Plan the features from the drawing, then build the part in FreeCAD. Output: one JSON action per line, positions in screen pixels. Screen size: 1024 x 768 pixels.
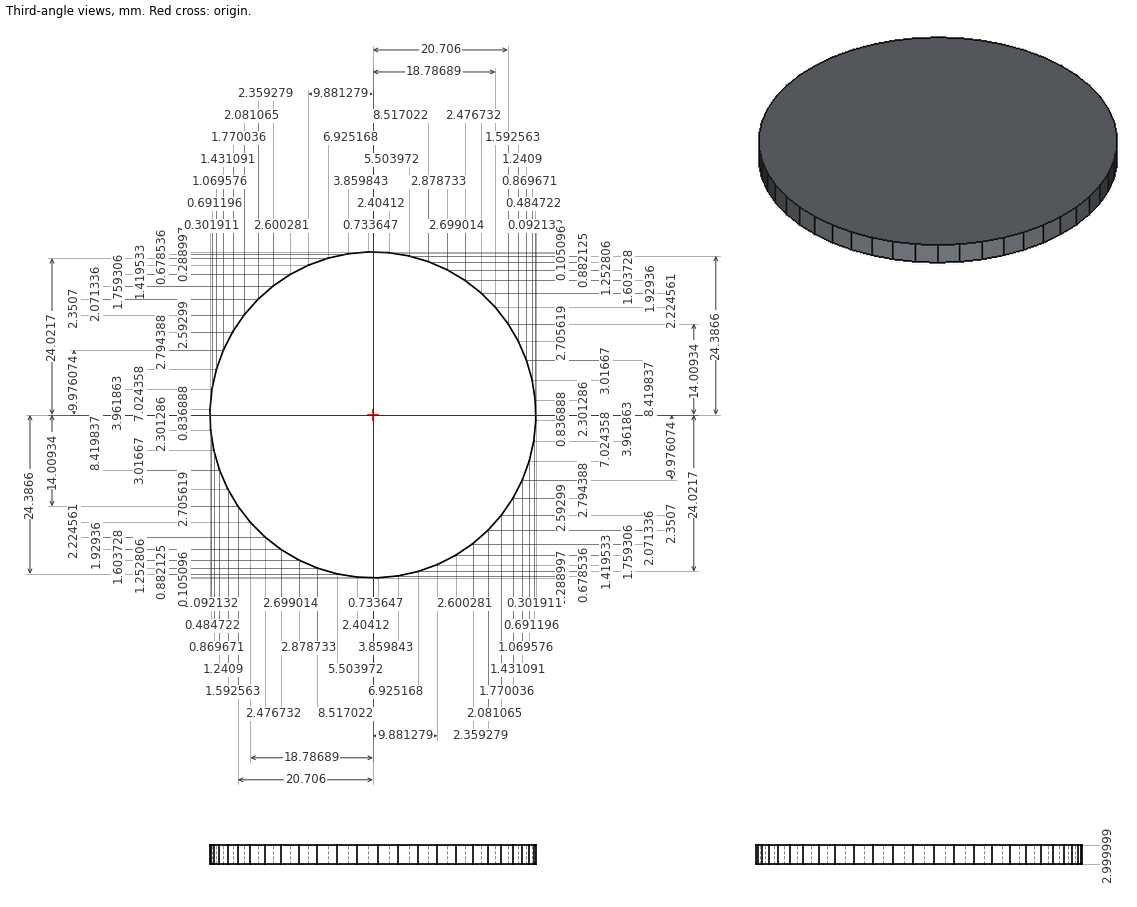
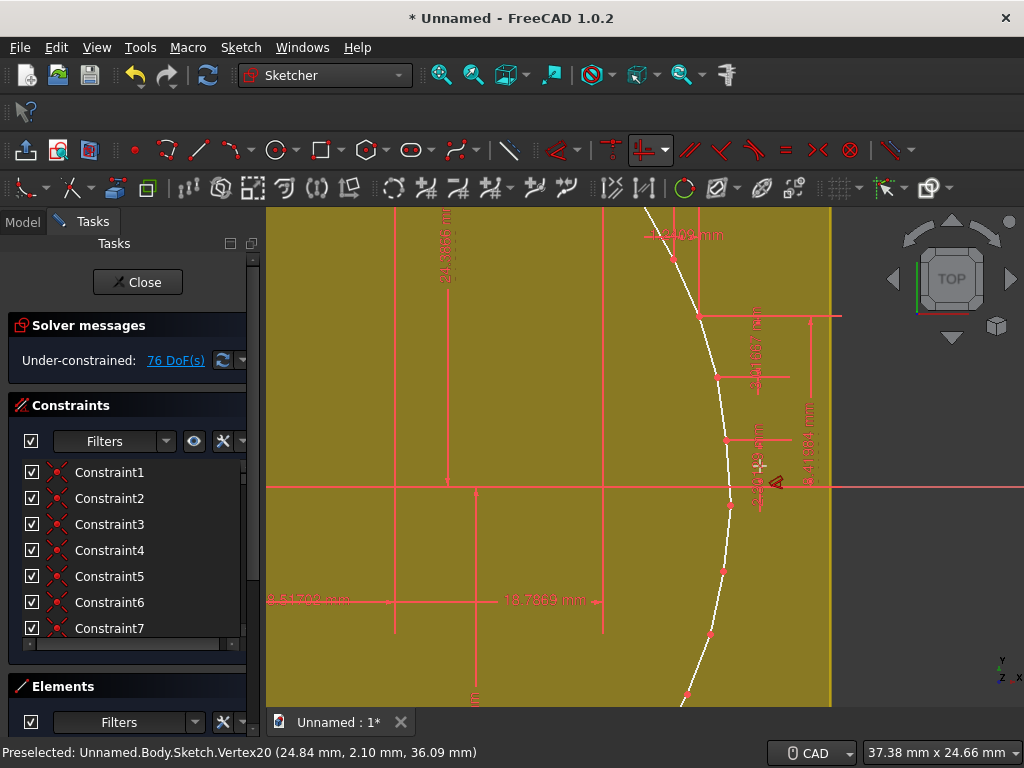
{"action": "scroll", "coordinate": [731, 505], "scroll_direction": "up", "scroll_amount": 5}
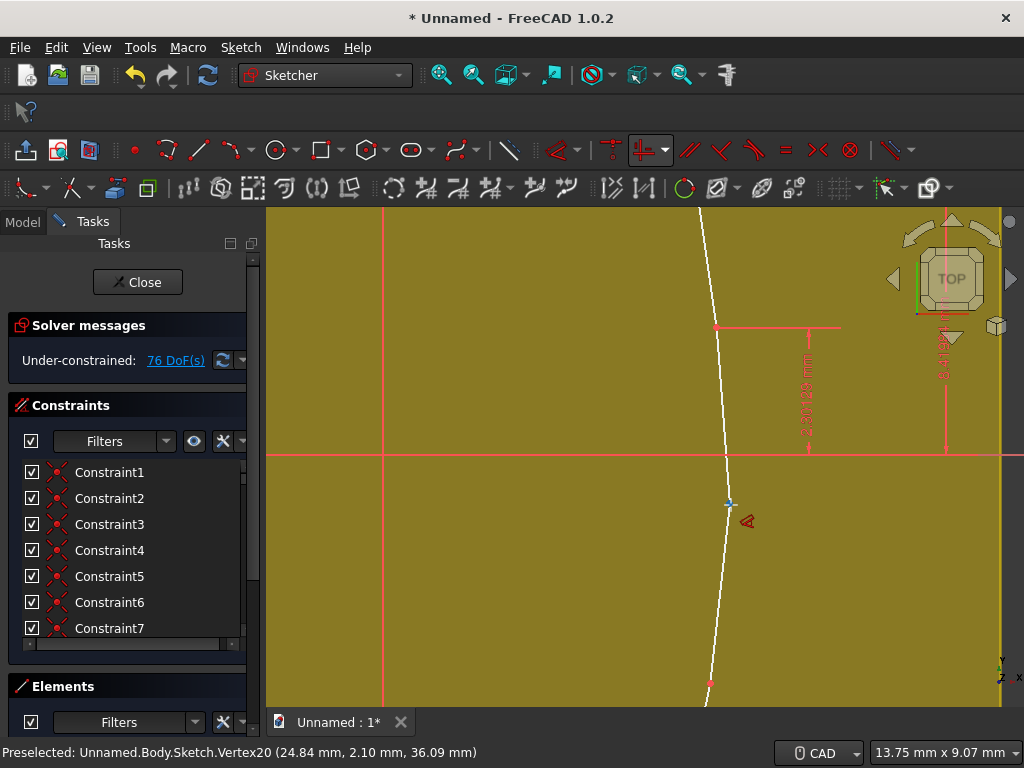
{"action": "left_click", "coordinate": [730, 504]}
{"action": "left_click", "coordinate": [764, 479]}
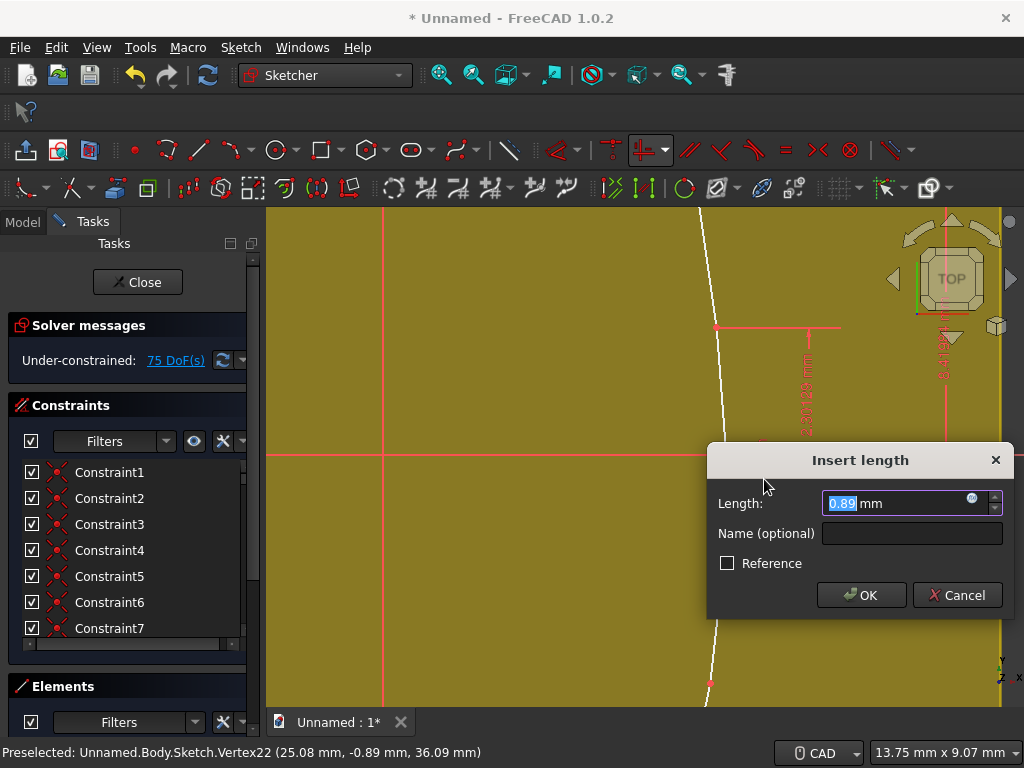
{"action": "type", "text": "0.836888"}
{"action": "key", "text": "Return"}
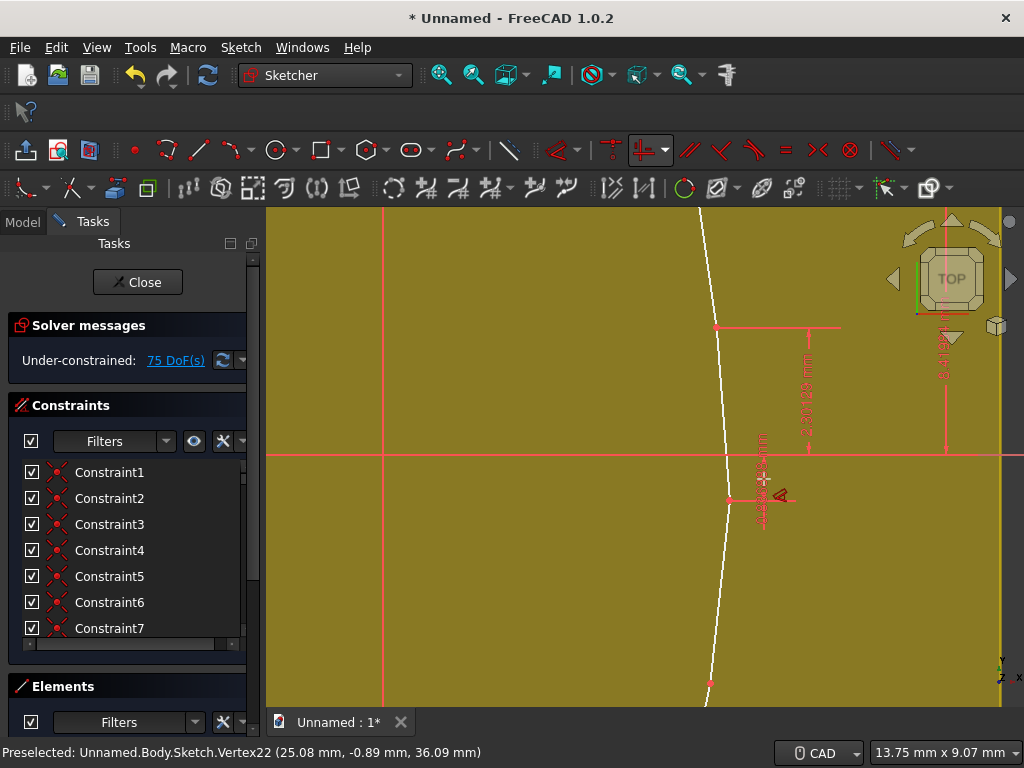
{"action": "scroll", "coordinate": [730, 457], "scroll_direction": "down", "scroll_amount": 11}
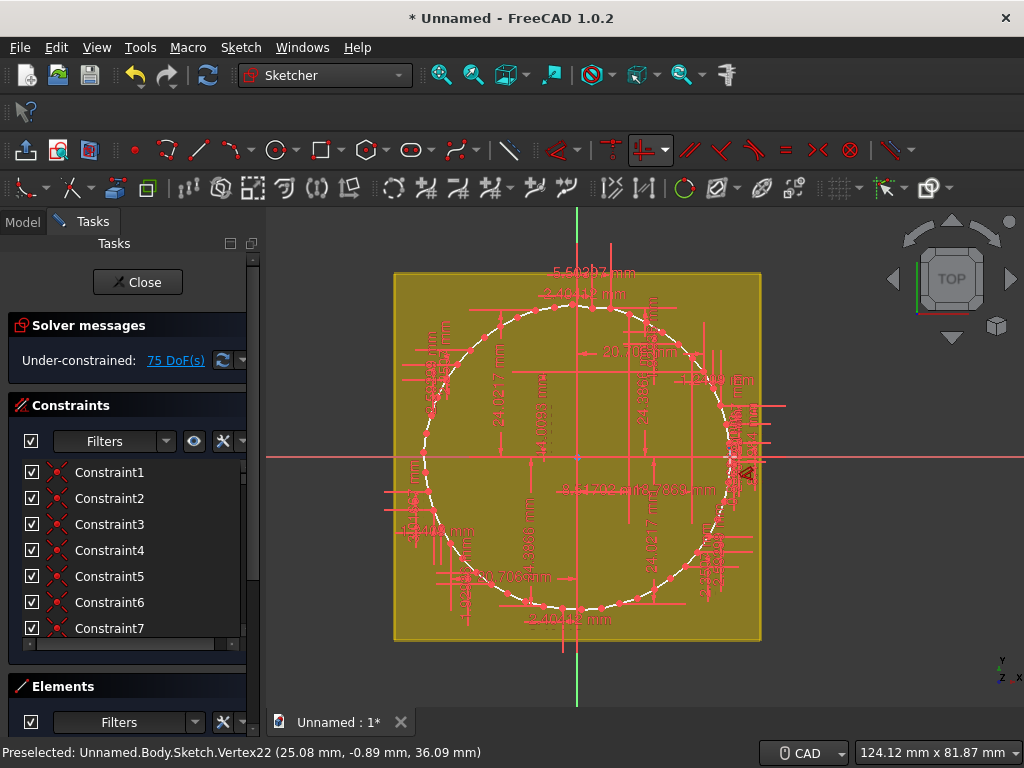
{"action": "scroll", "coordinate": [728, 483], "scroll_direction": "up", "scroll_amount": 3}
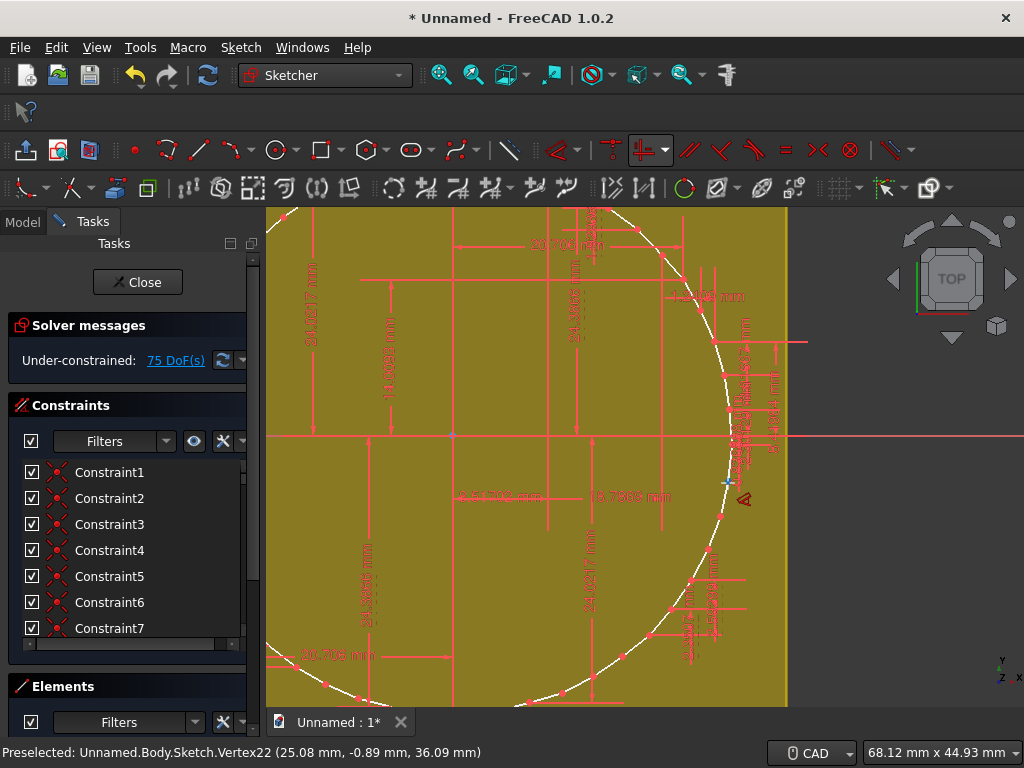
{"action": "left_click", "coordinate": [728, 482]}
{"action": "left_click", "coordinate": [762, 469]}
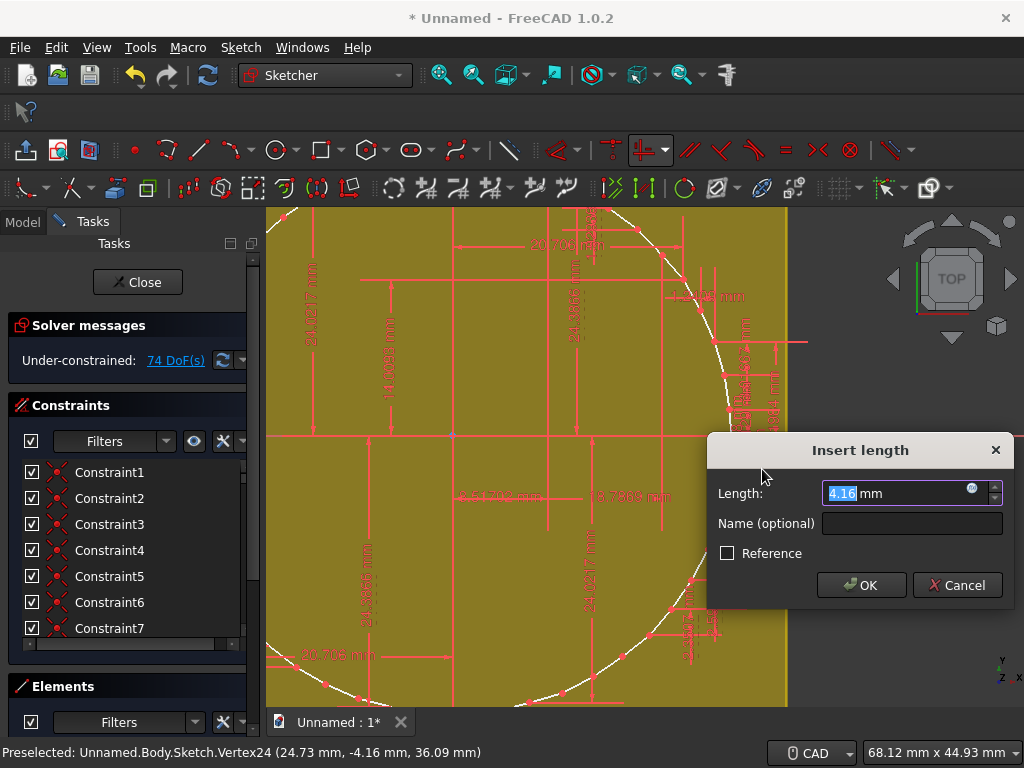
{"action": "type", "text": "3.961863"}
{"action": "key", "text": "Return"}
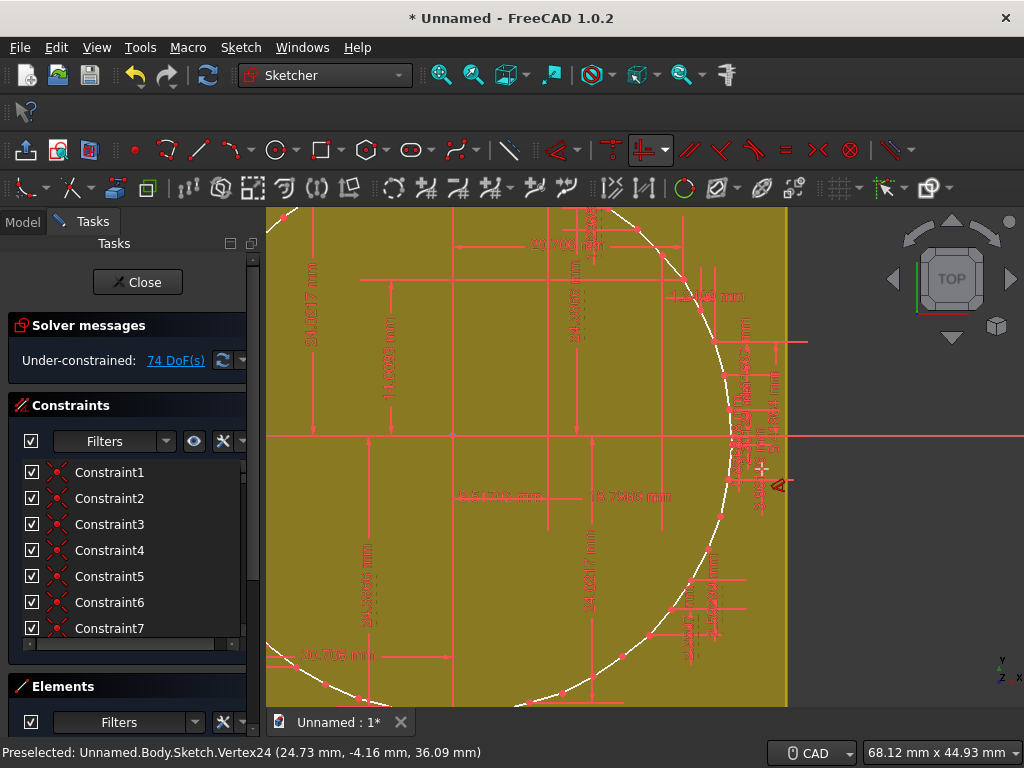
{"action": "left_click", "coordinate": [721, 516]}
{"action": "left_click", "coordinate": [755, 495]}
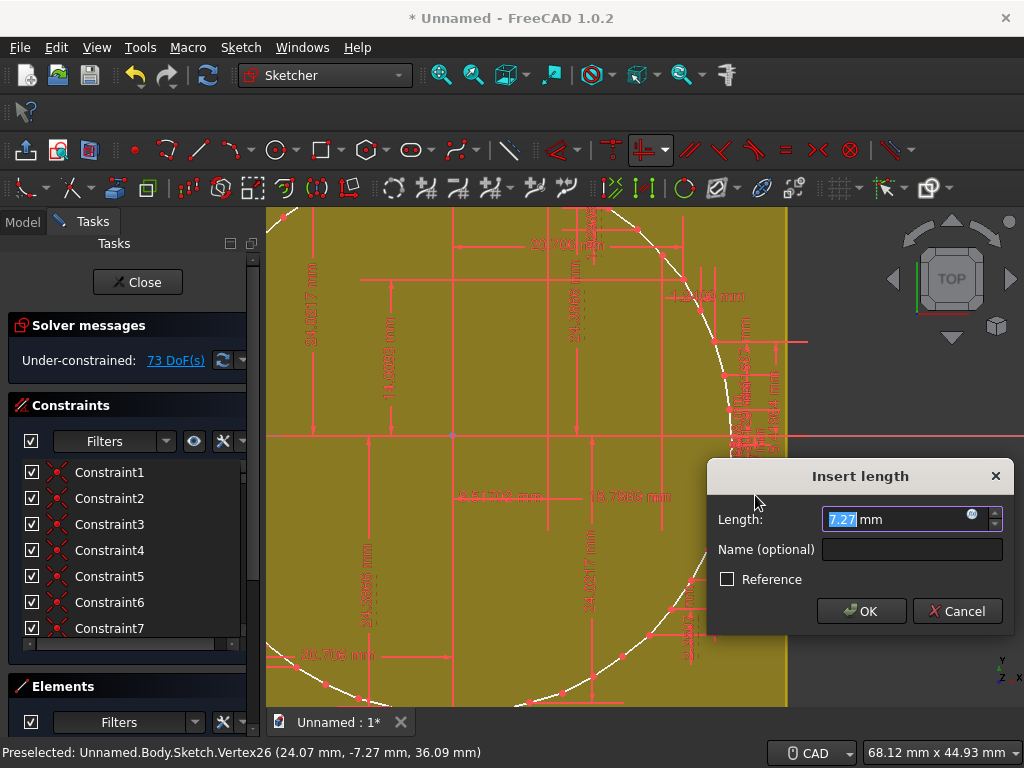
{"action": "type", "text": "7.024358"}
{"action": "key", "text": "Return"}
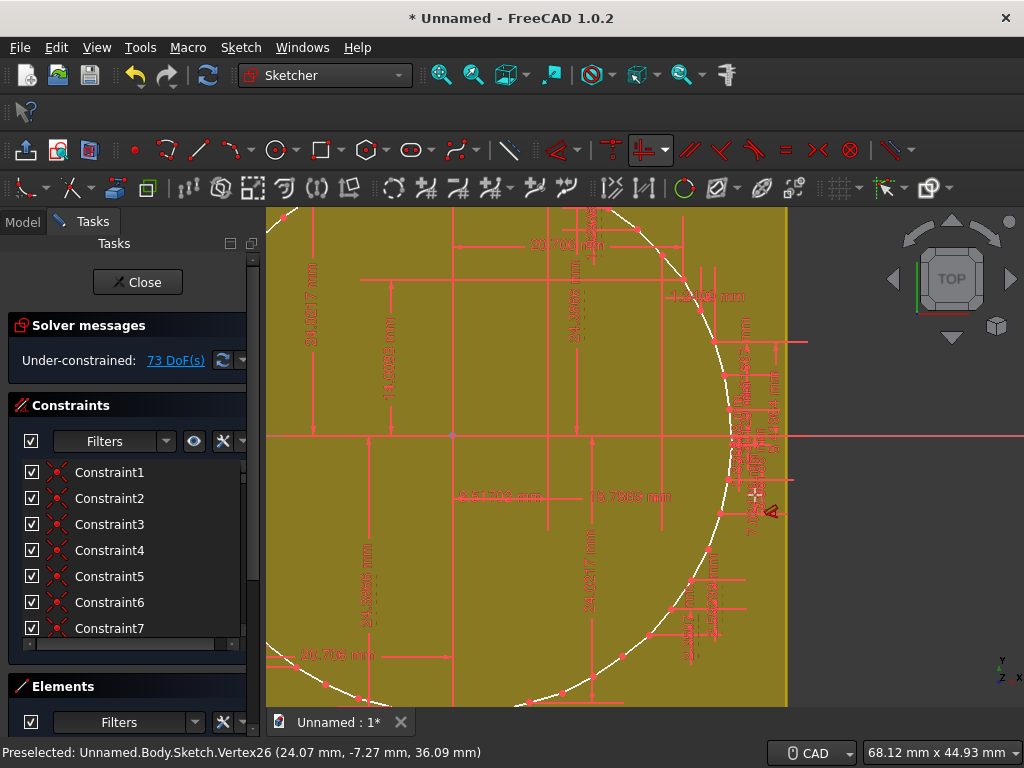
{"action": "left_click", "coordinate": [708, 549]}
{"action": "left_click", "coordinate": [742, 519]}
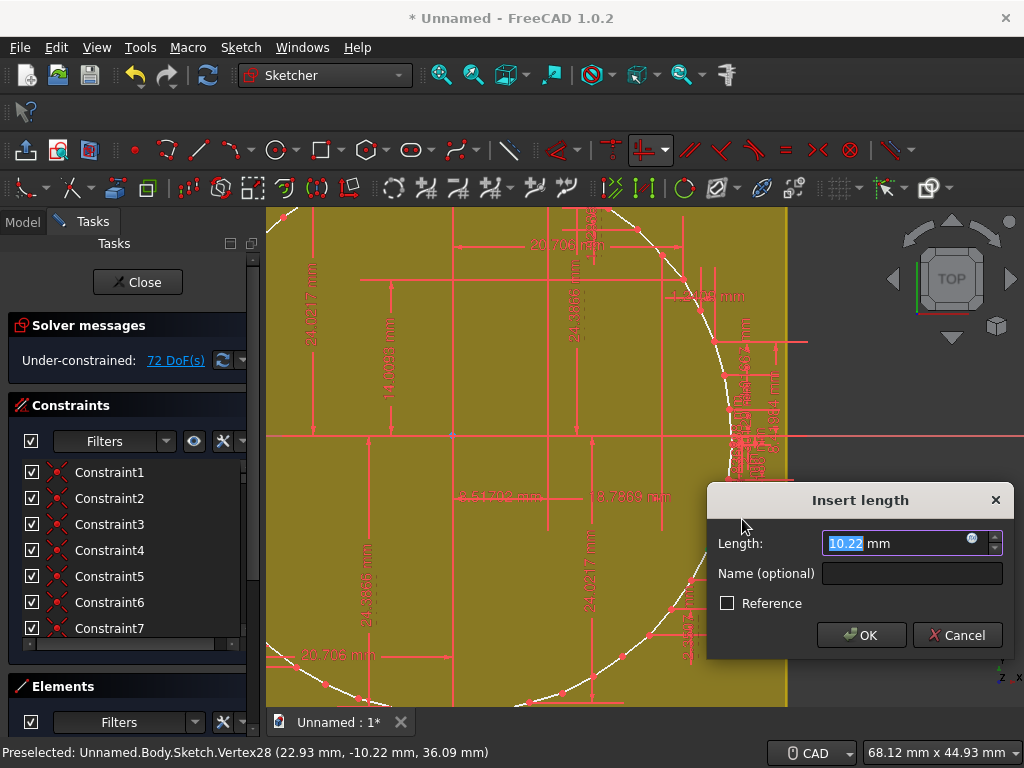
{"action": "type", "text": "9.976074"}
{"action": "key", "text": "Return"}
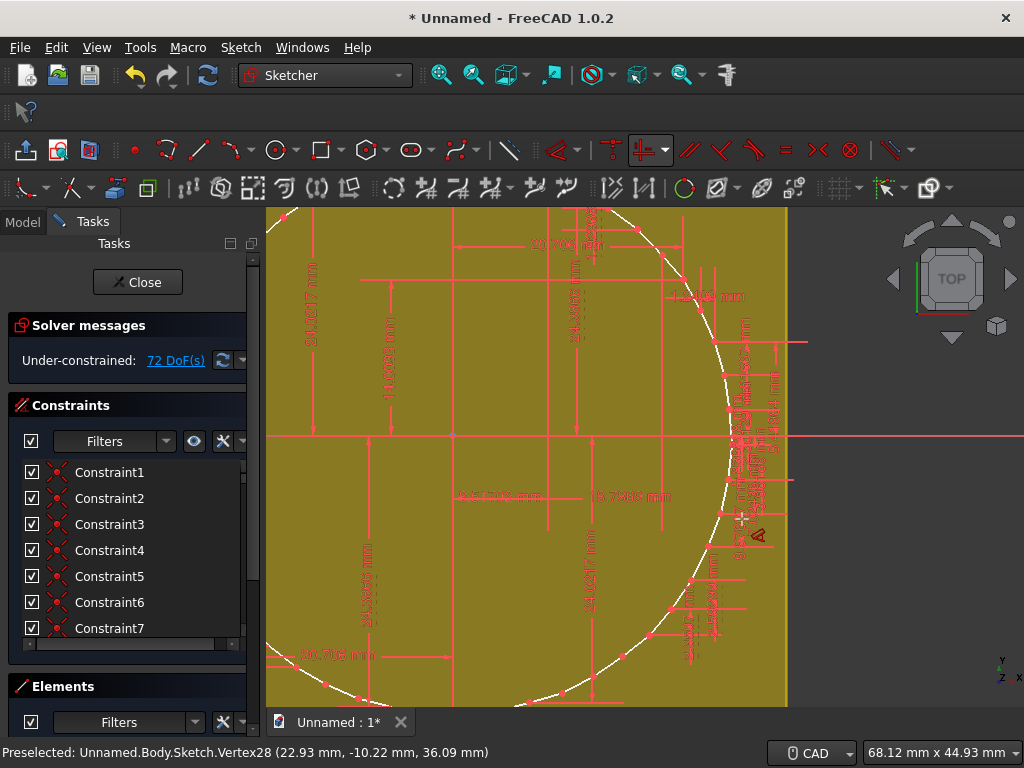
{"action": "scroll", "coordinate": [727, 483], "scroll_direction": "down", "scroll_amount": 3}